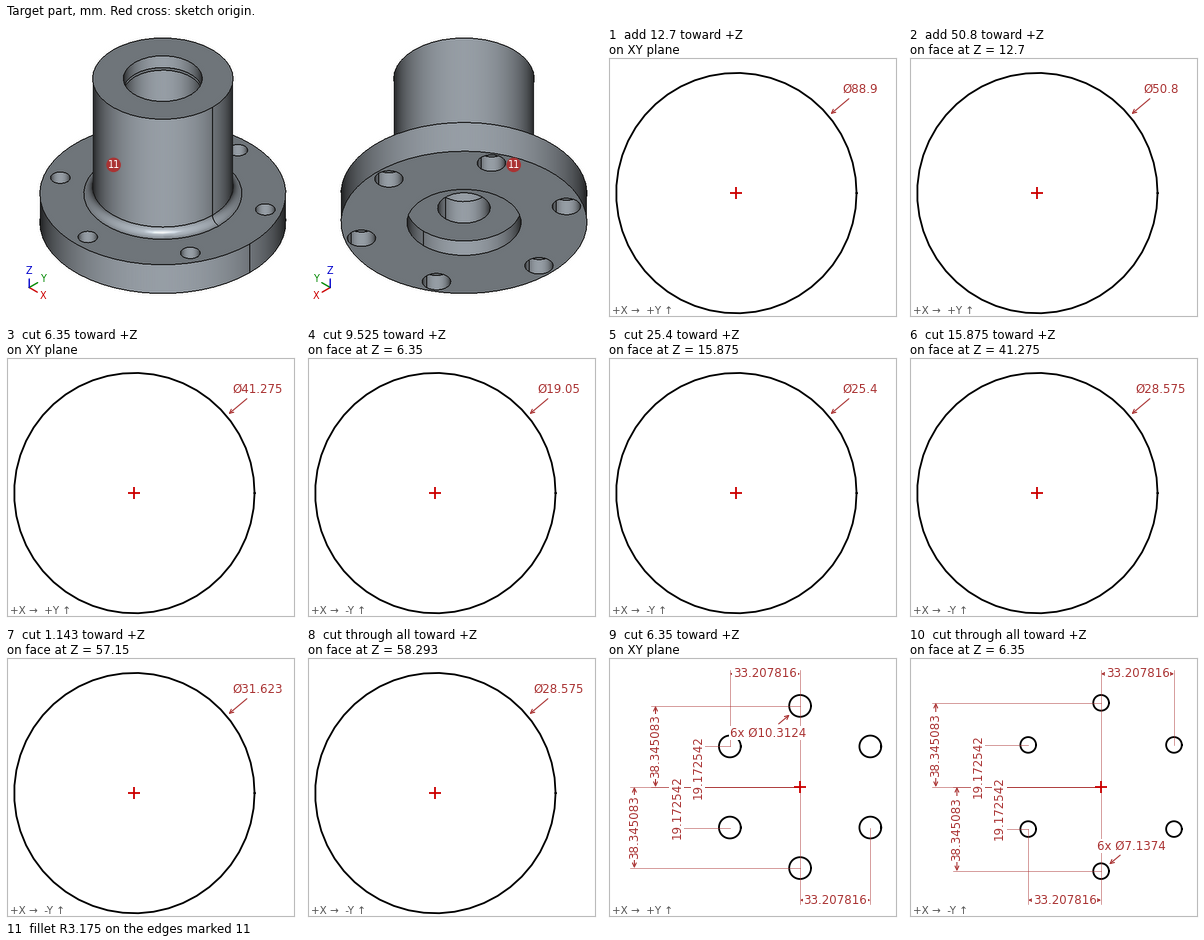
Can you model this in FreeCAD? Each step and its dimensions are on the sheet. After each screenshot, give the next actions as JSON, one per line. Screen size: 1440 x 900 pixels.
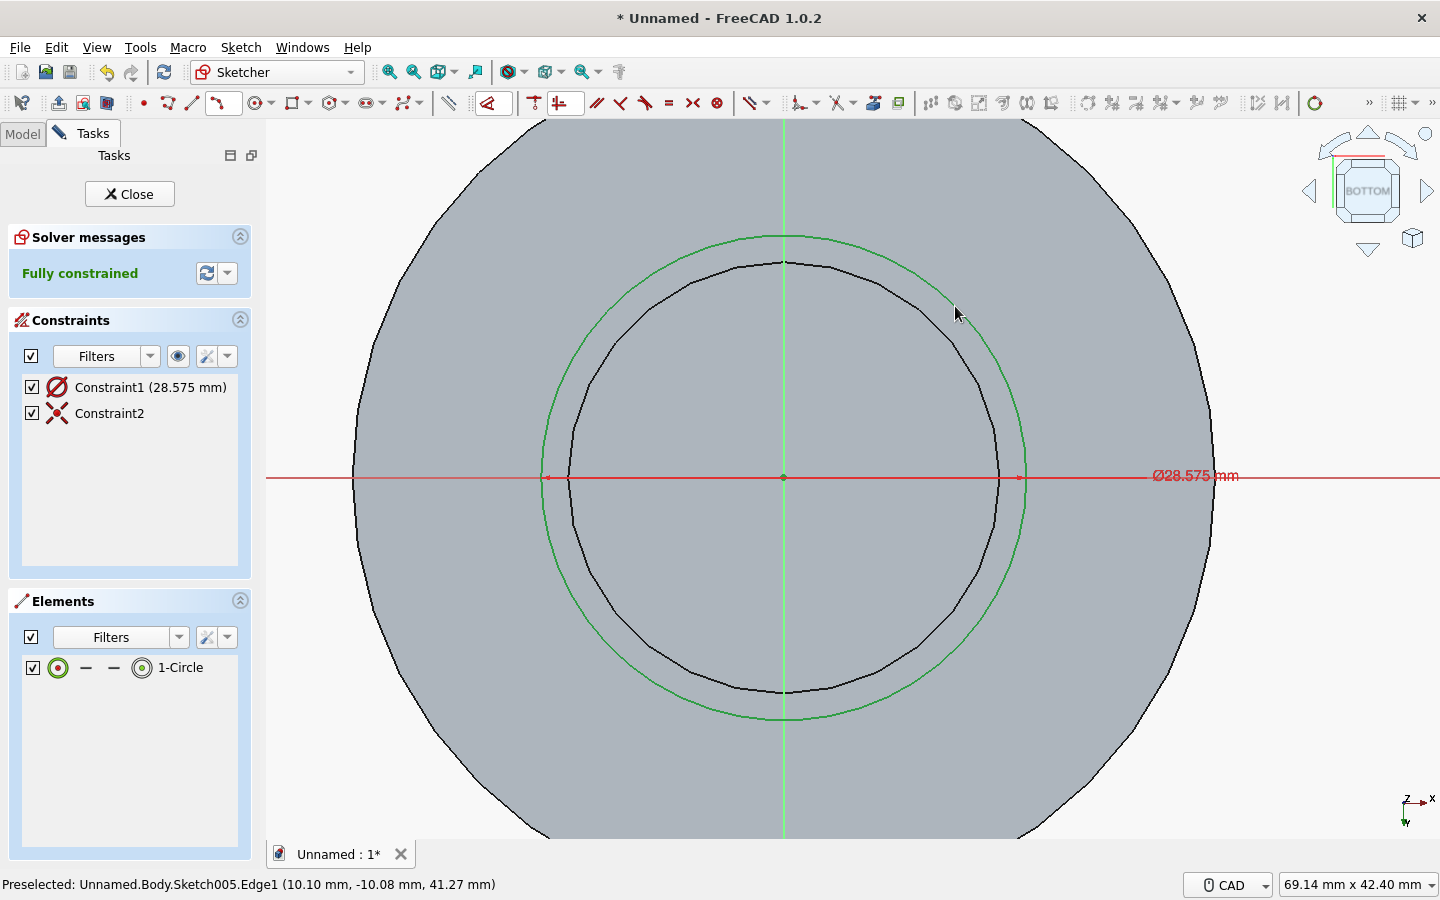
{"action": "left_click", "coordinate": [130, 194]}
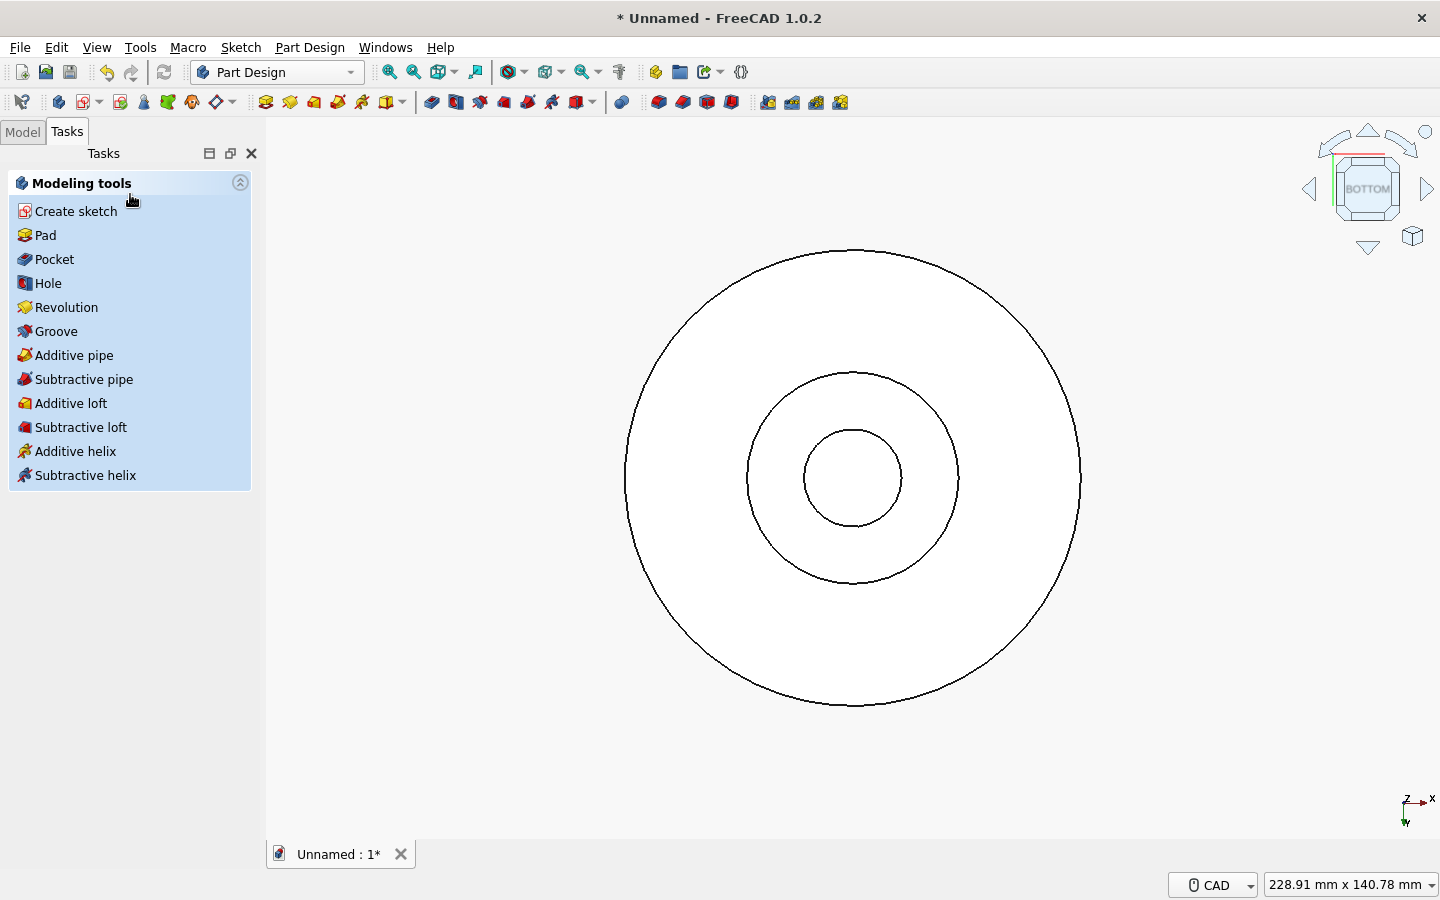
{"action": "left_click", "coordinate": [432, 102]}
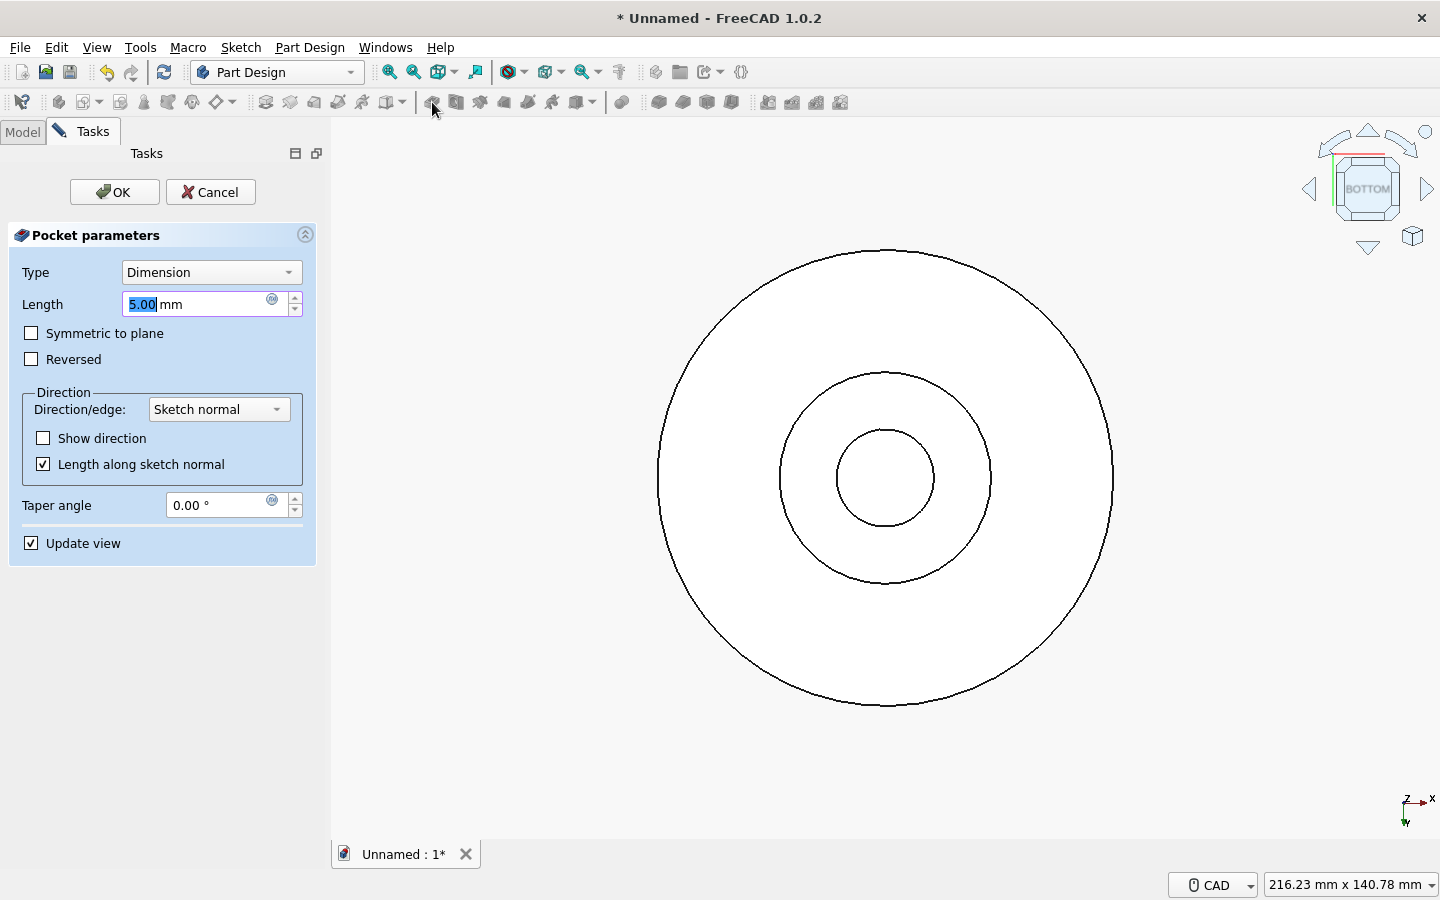
{"action": "type", "text": "15.875"}
{"action": "key", "text": "Tab"}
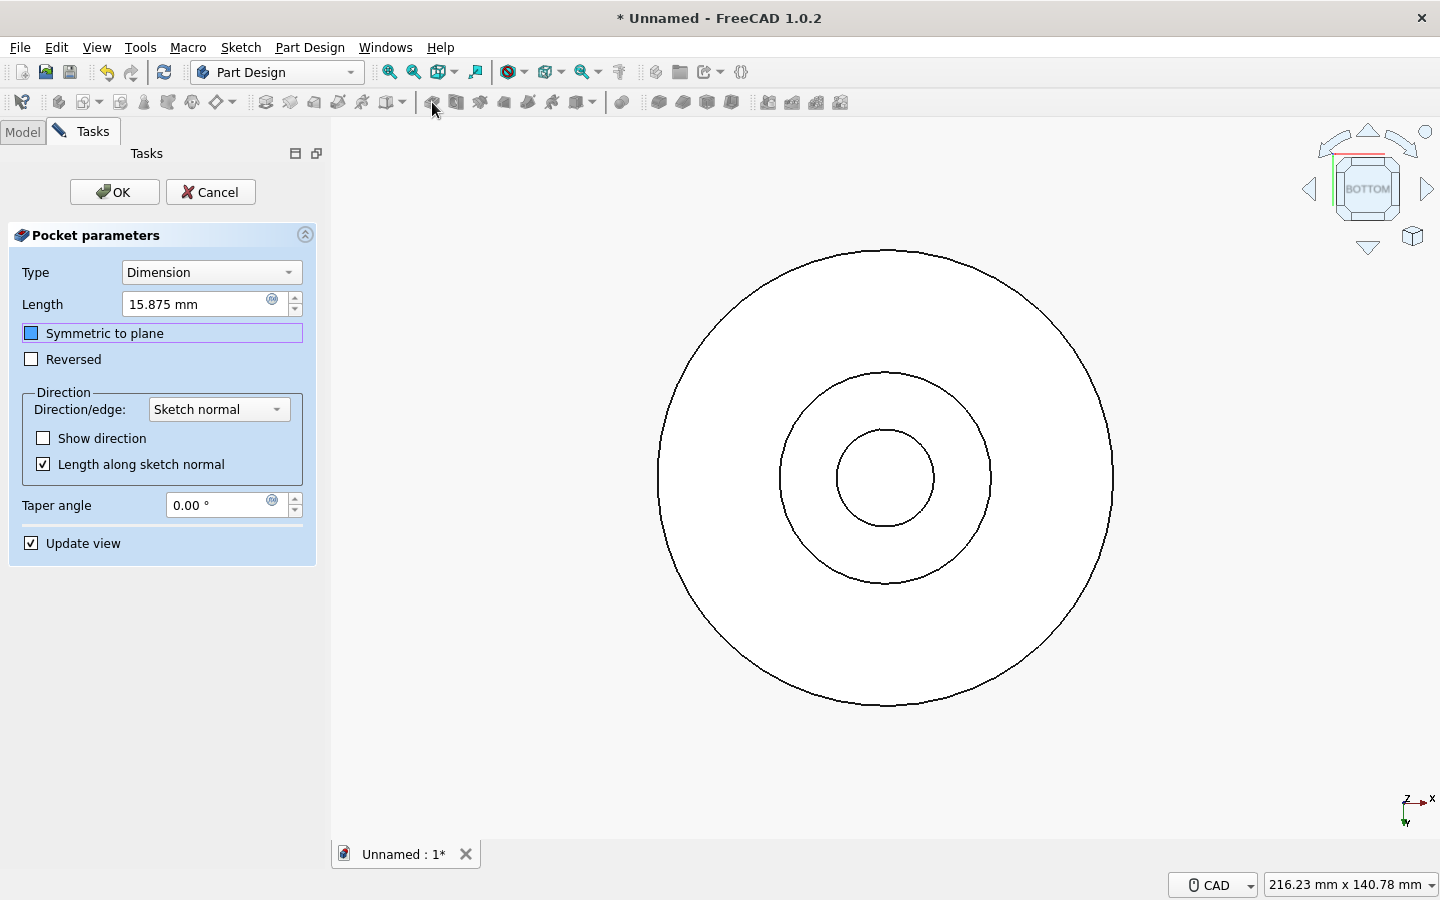
{"action": "left_click", "coordinate": [115, 192]}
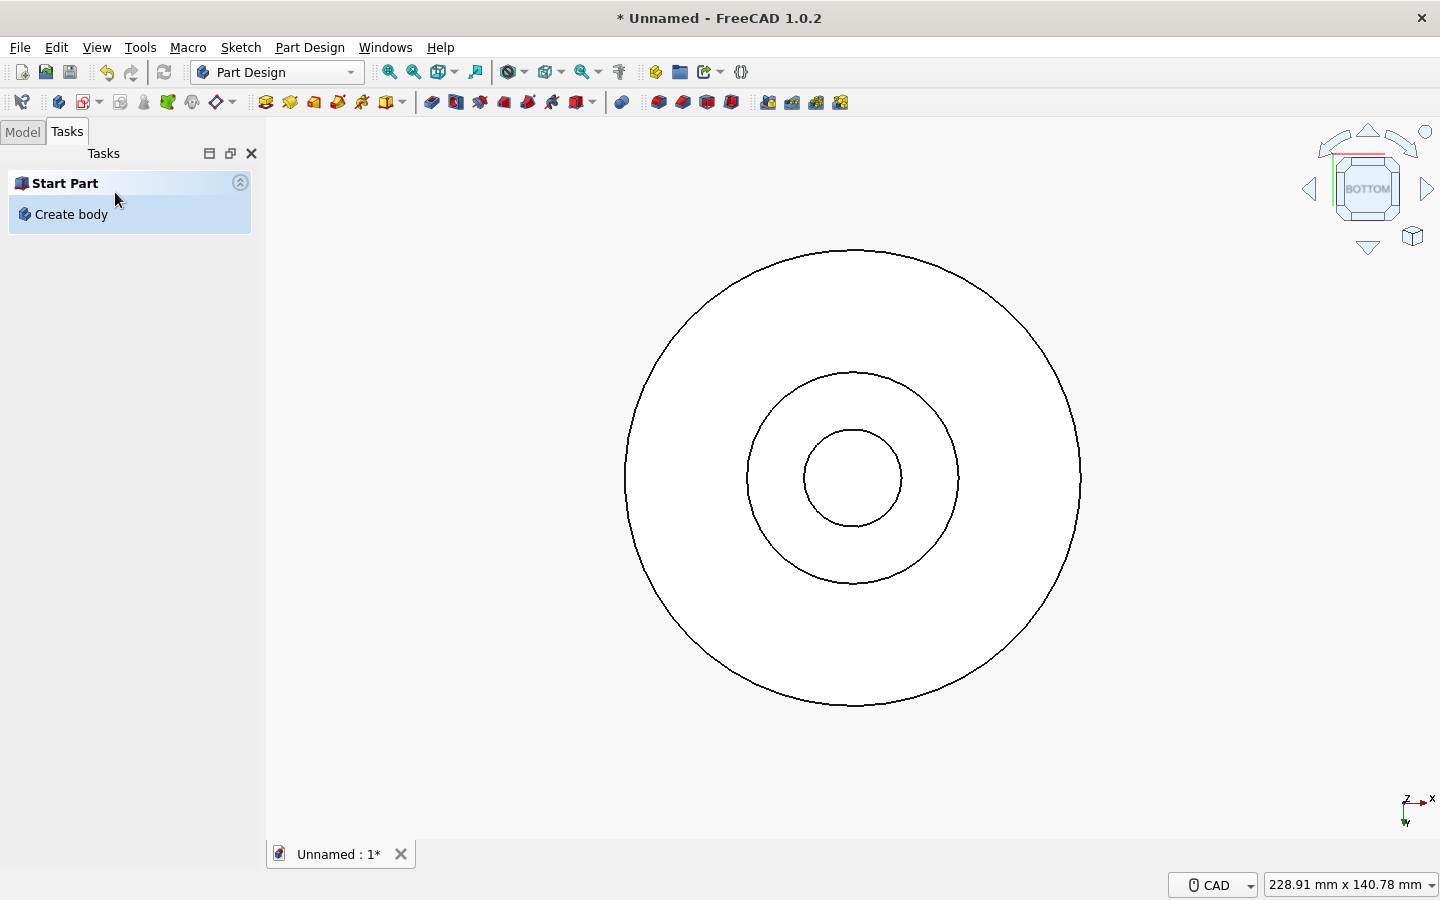
{"action": "left_click", "coordinate": [853, 477]}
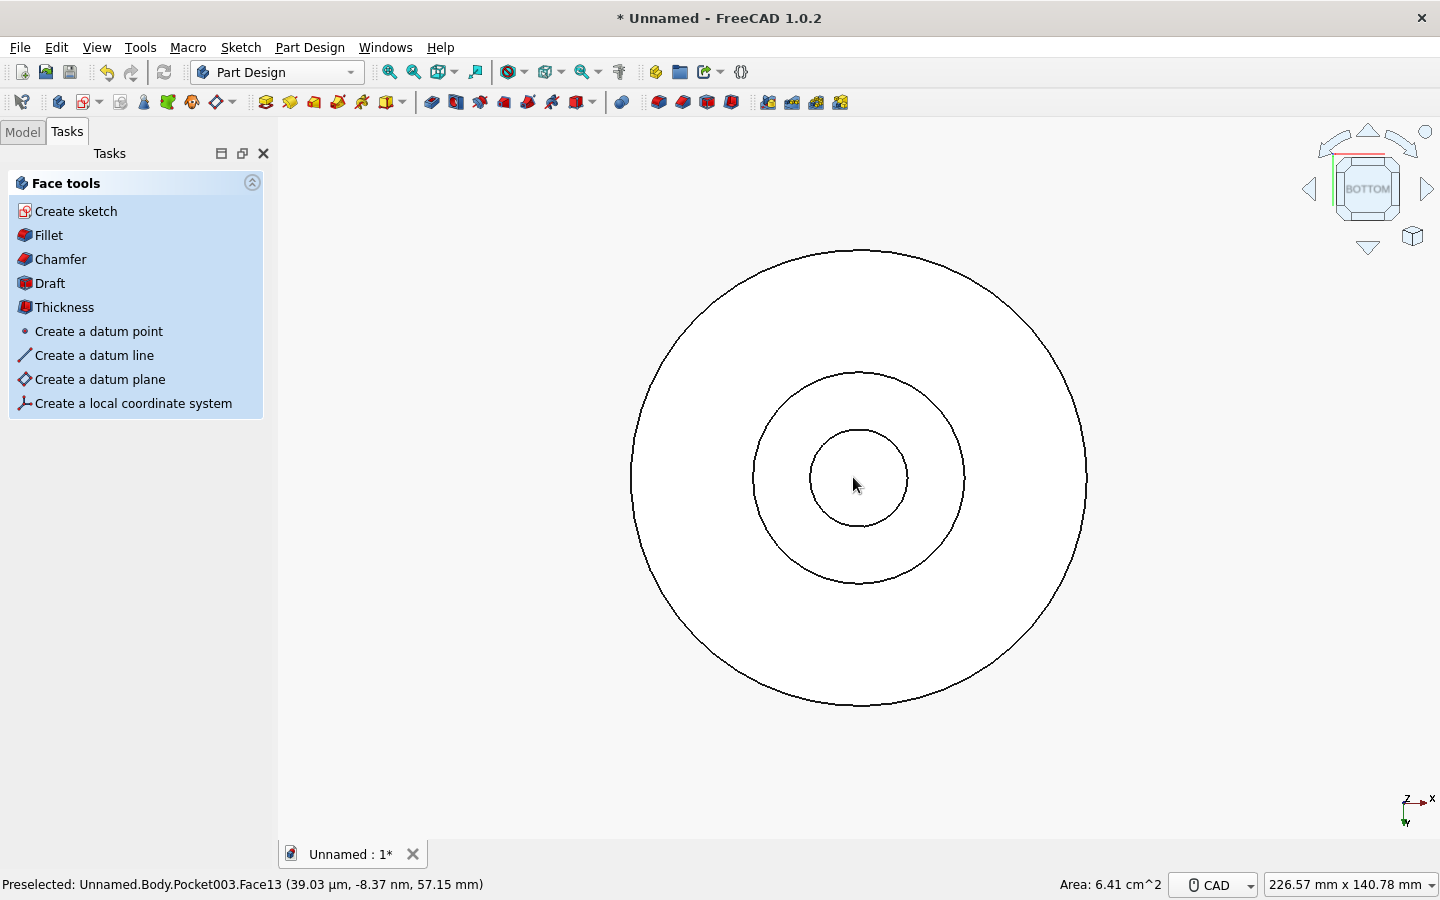
{"action": "left_click", "coordinate": [84, 102]}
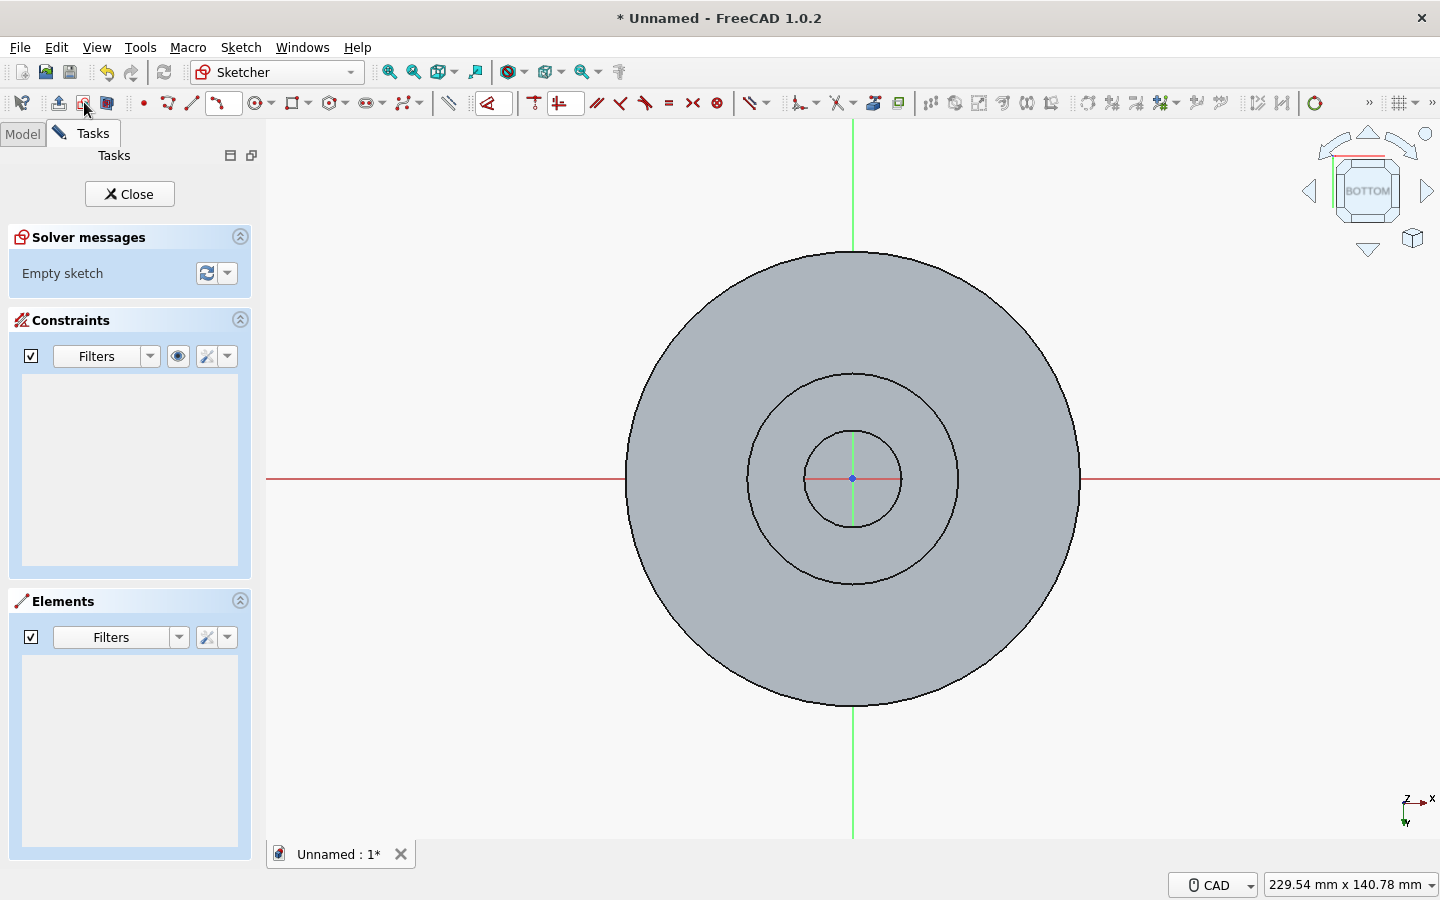
{"action": "scroll", "coordinate": [893, 479], "scroll_direction": "up", "scroll_amount": 5}